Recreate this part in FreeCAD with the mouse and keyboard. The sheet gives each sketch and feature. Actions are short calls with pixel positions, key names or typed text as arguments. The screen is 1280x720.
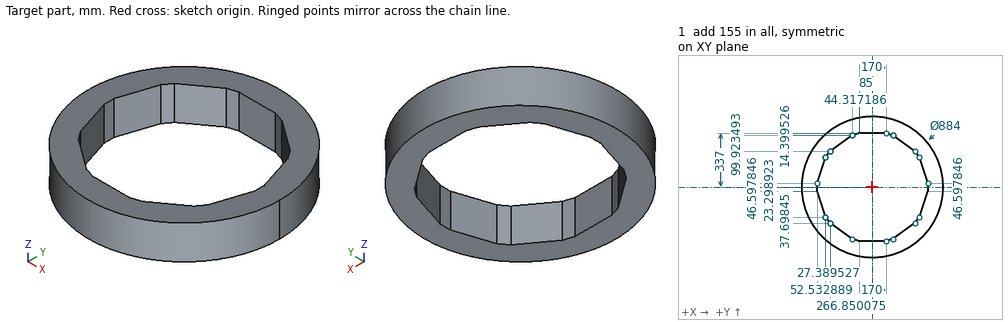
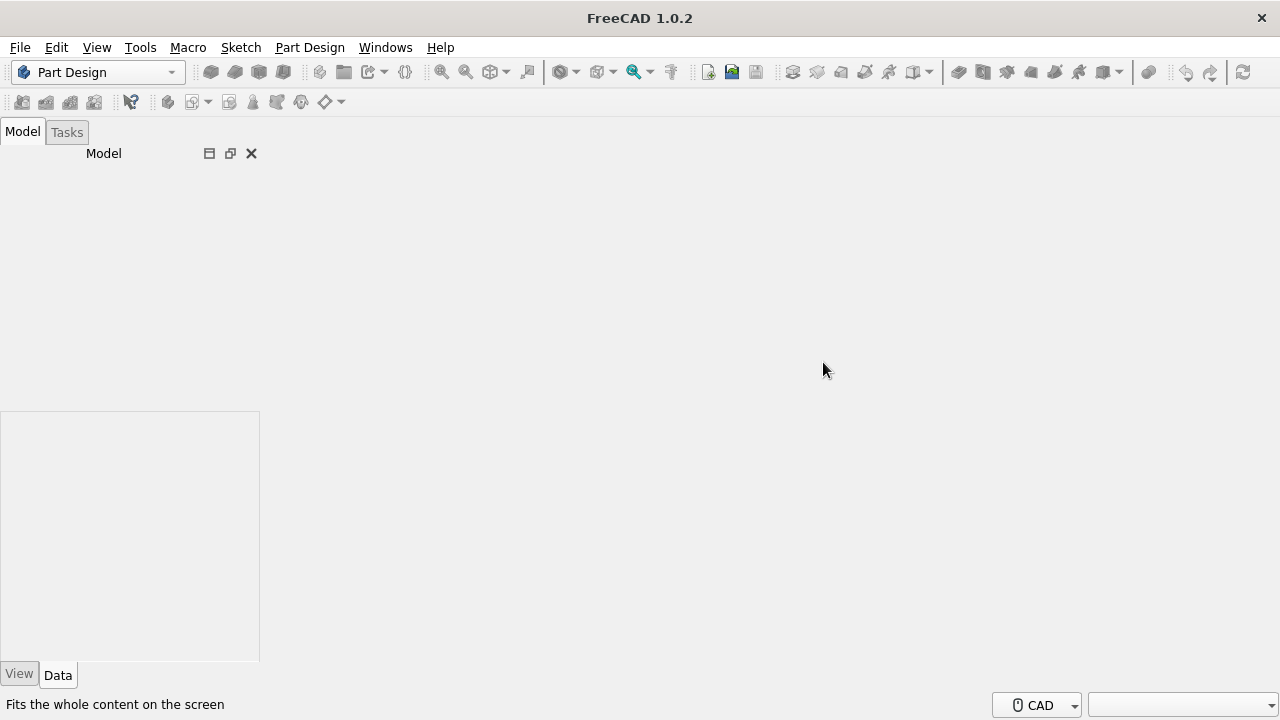
key(ctrl+n)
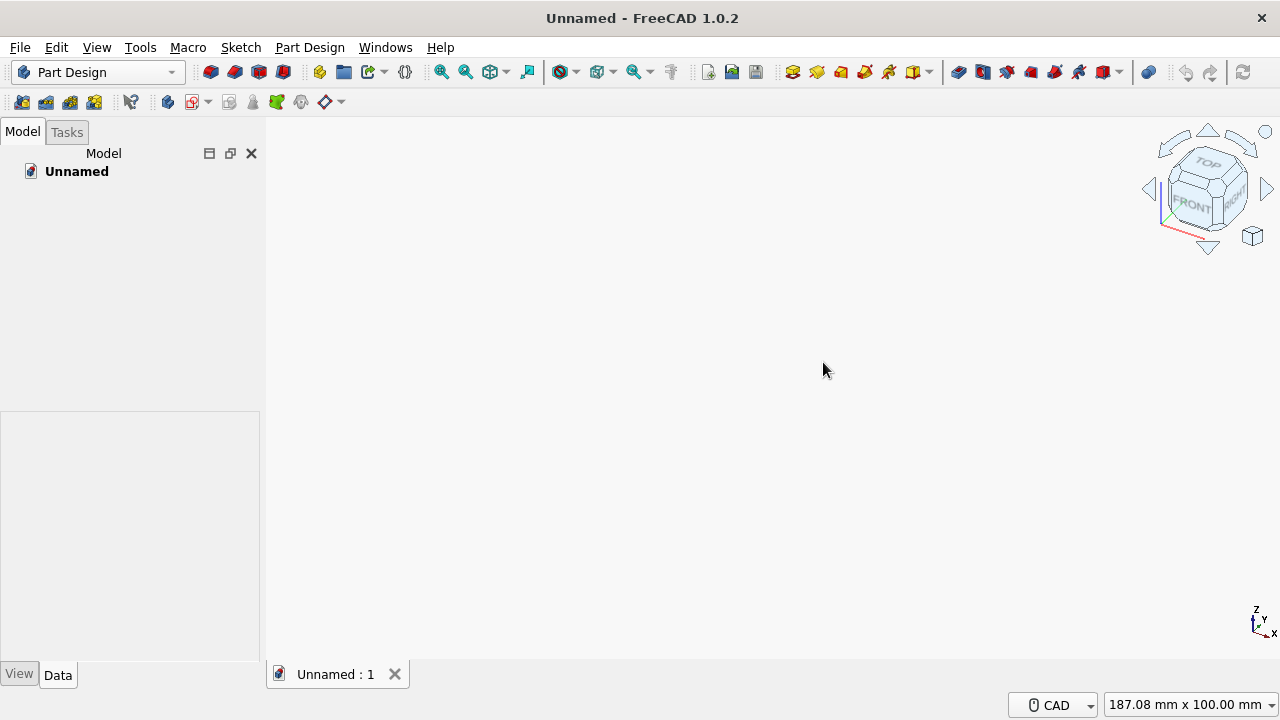
click(192, 102)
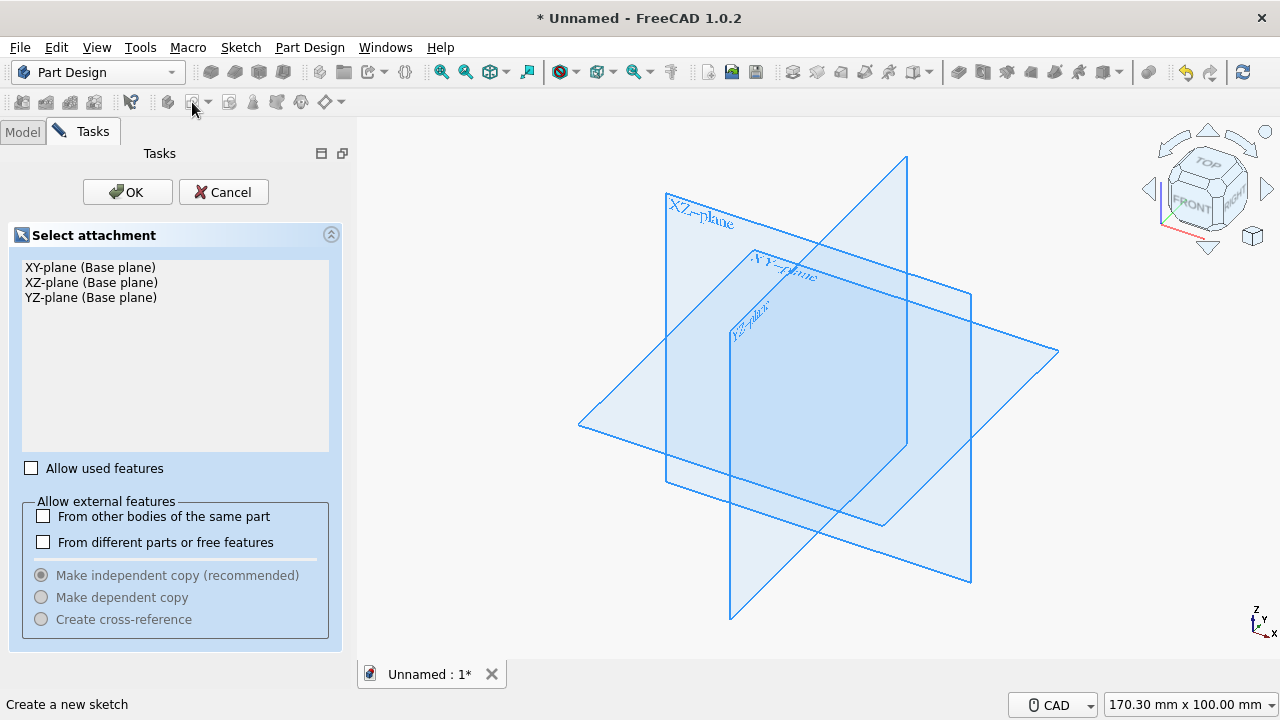
click(82, 268)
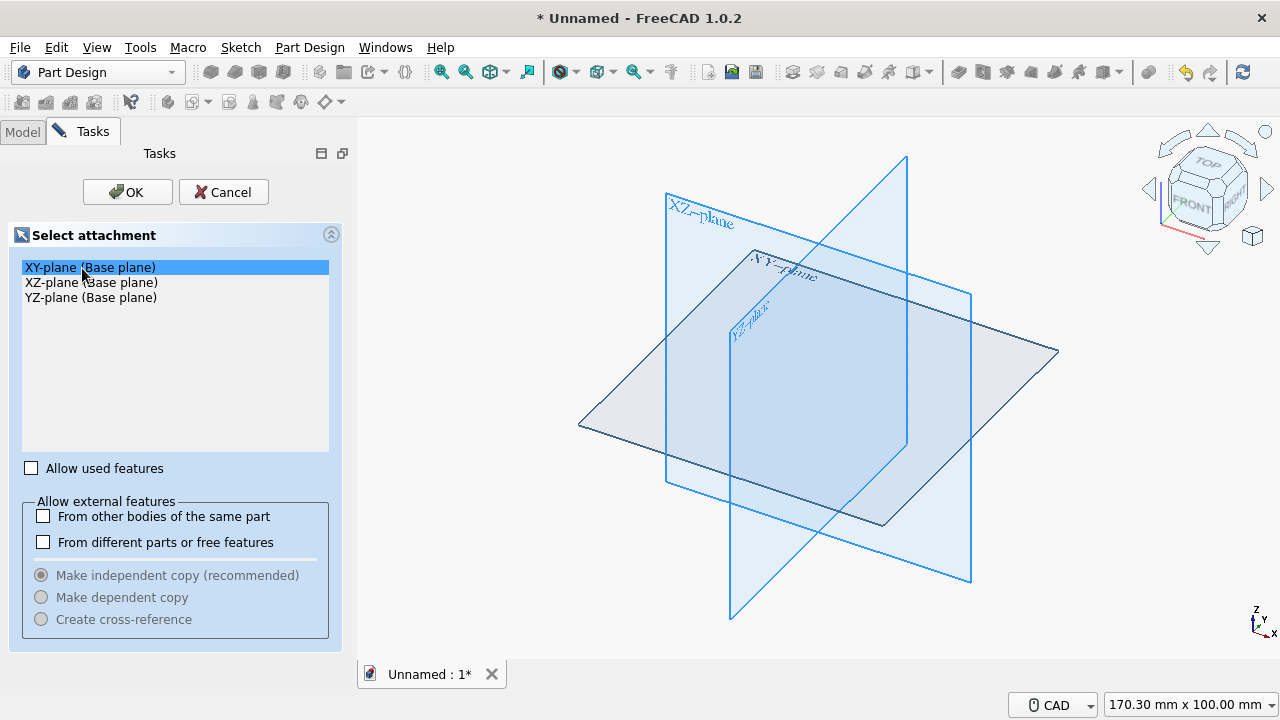
click(128, 192)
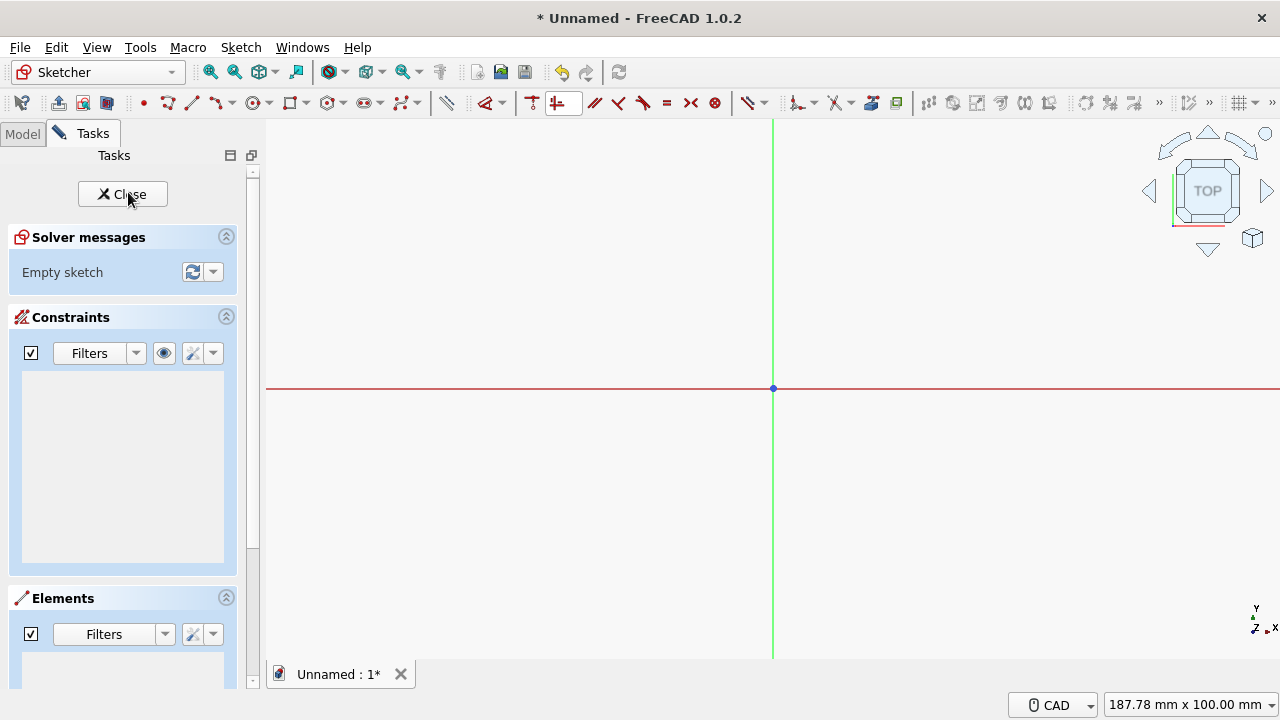
scroll(699, 389, down, 13)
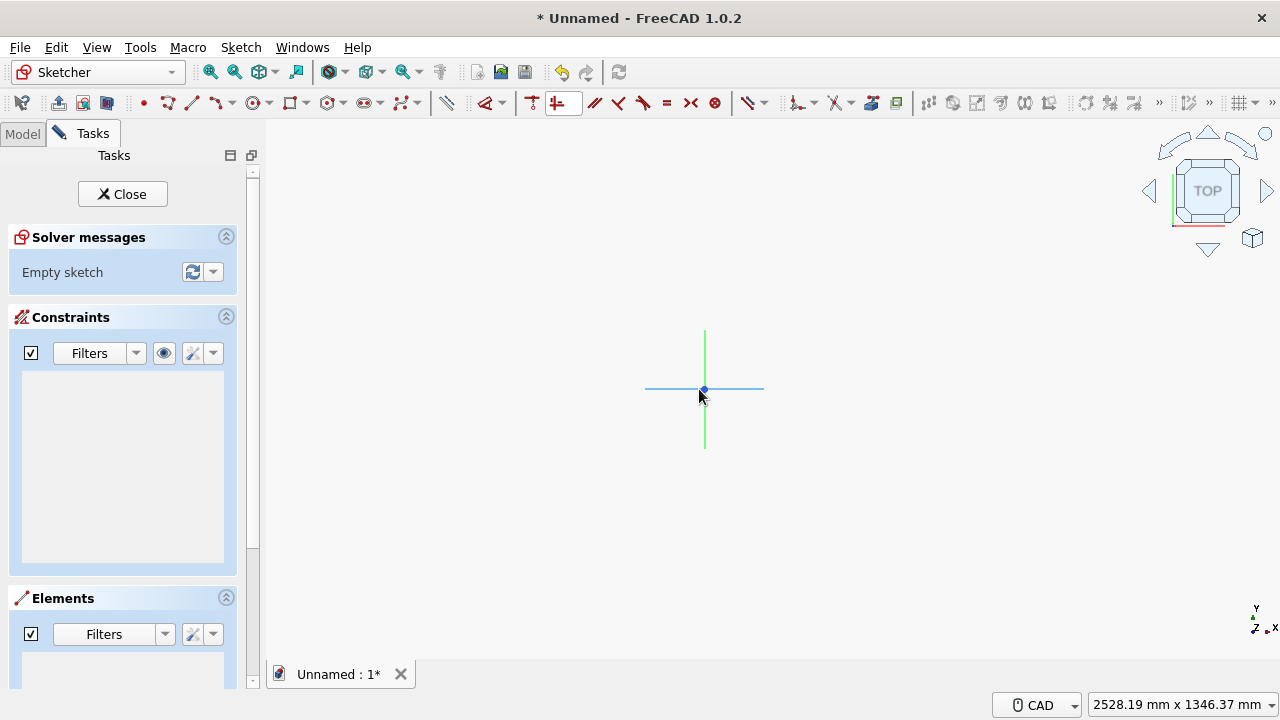
key(g)
key(m)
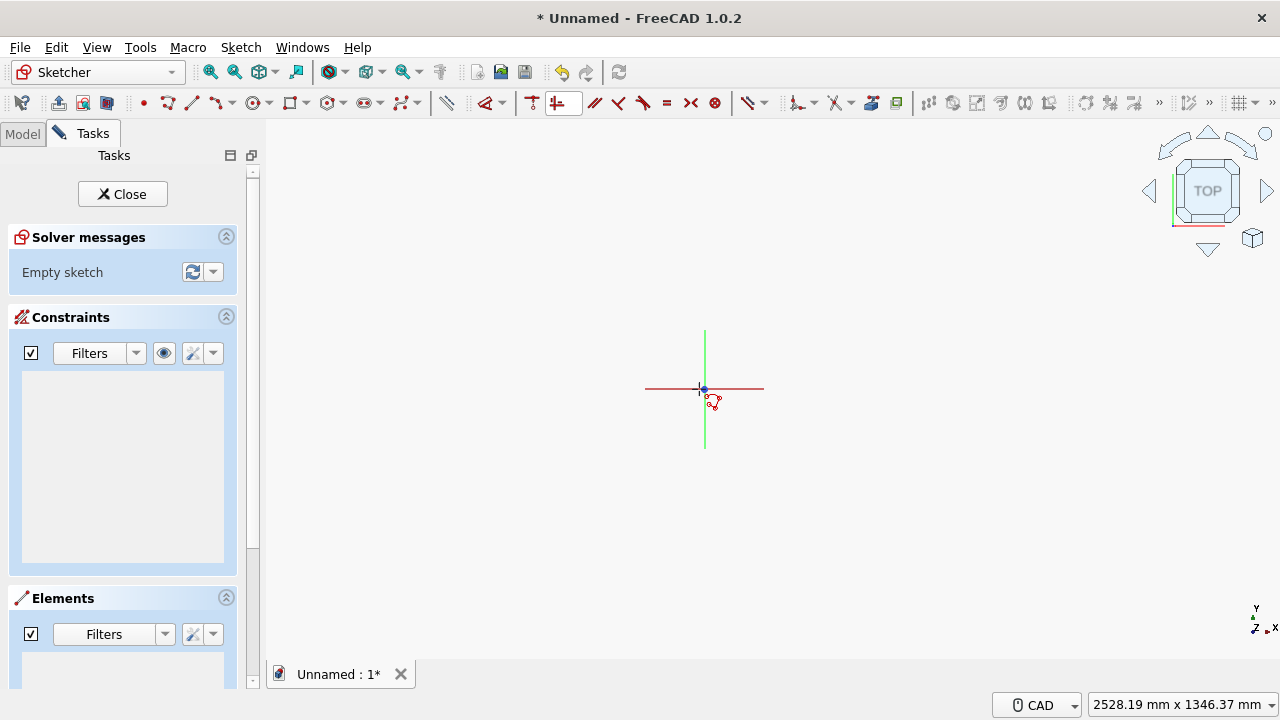
click(598, 479)
click(587, 464)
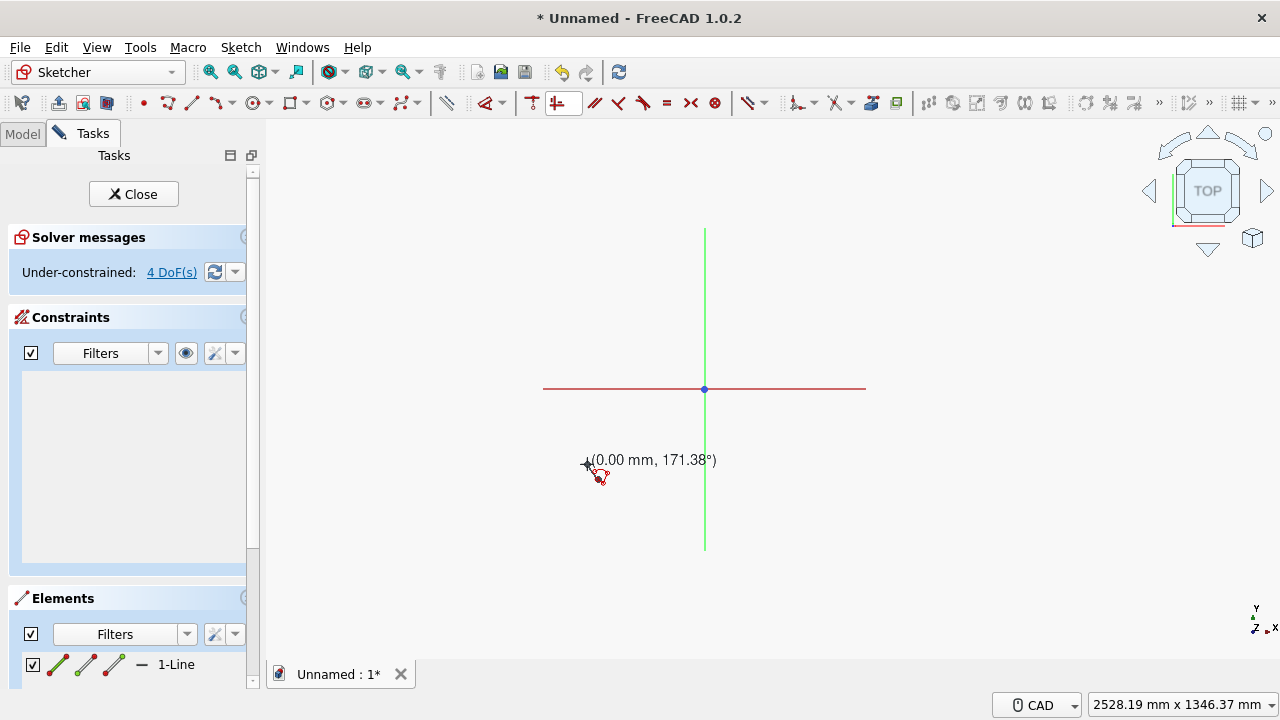
scroll(566, 399, up, 3)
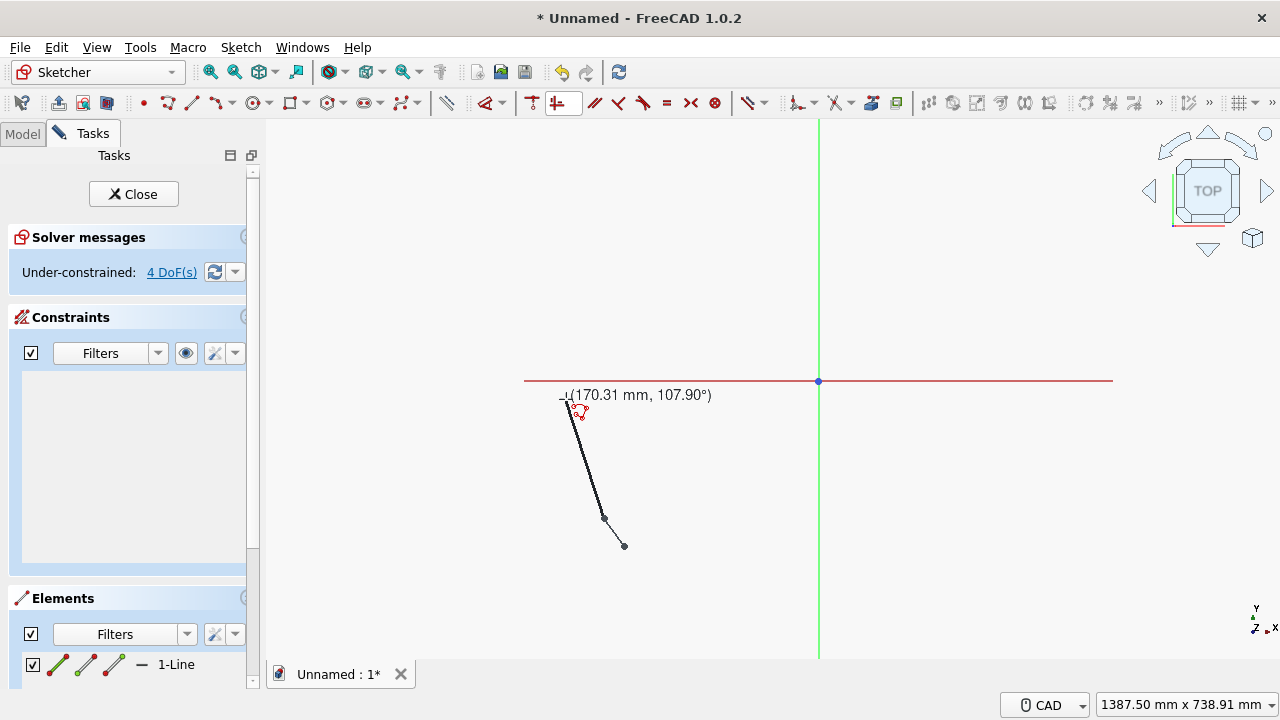
click(565, 398)
click(565, 364)
click(604, 246)
click(624, 218)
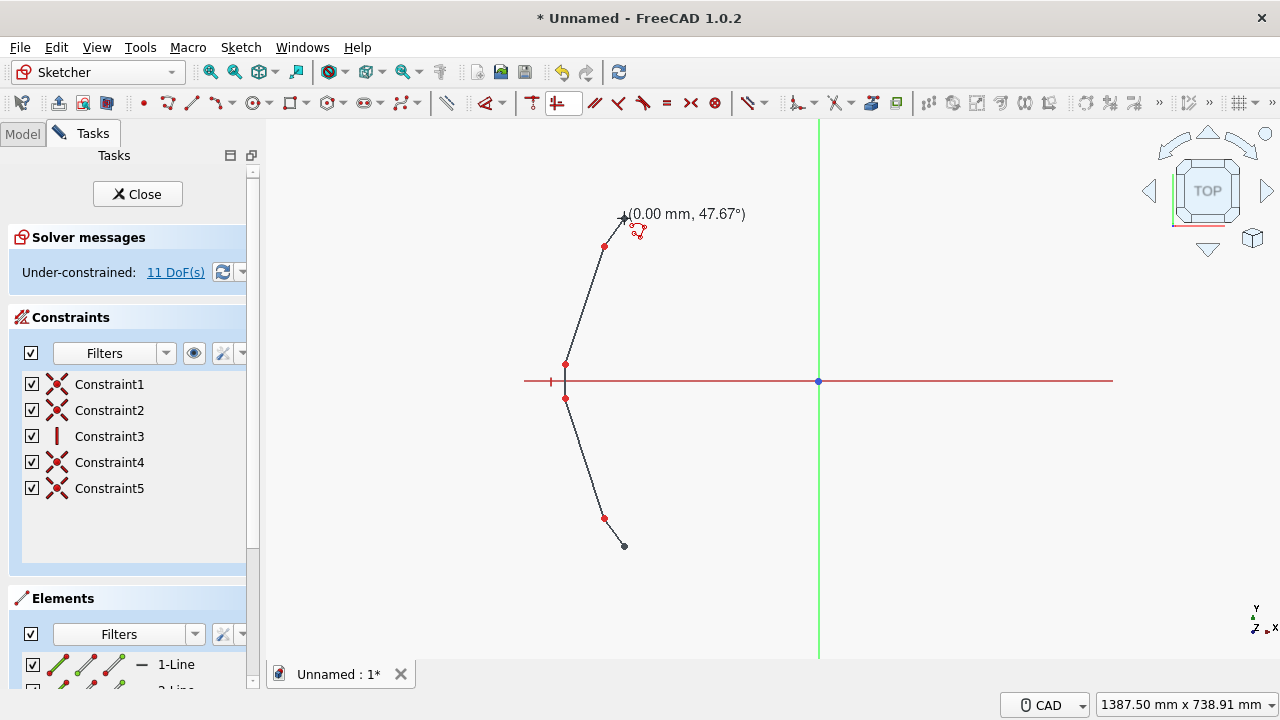
scroll(565, 398, down, 3)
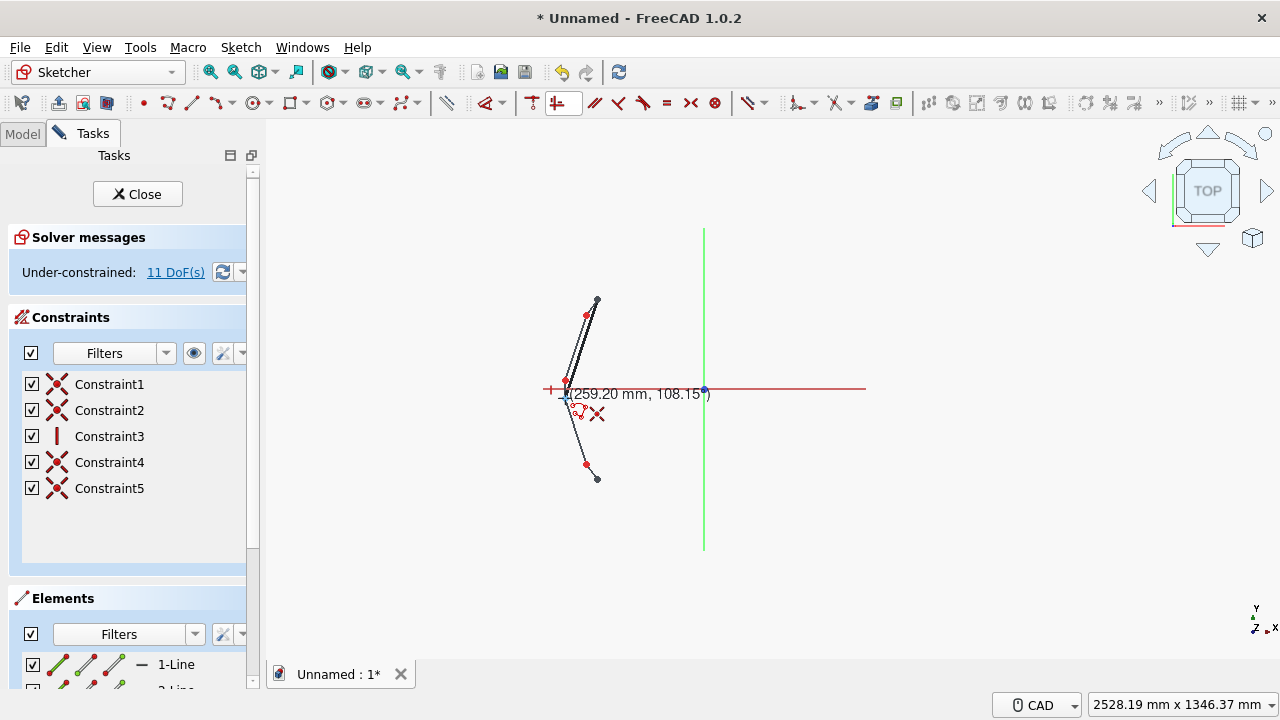
click(653, 260)
click(670, 254)
click(739, 254)
click(756, 260)
click(811, 300)
click(822, 315)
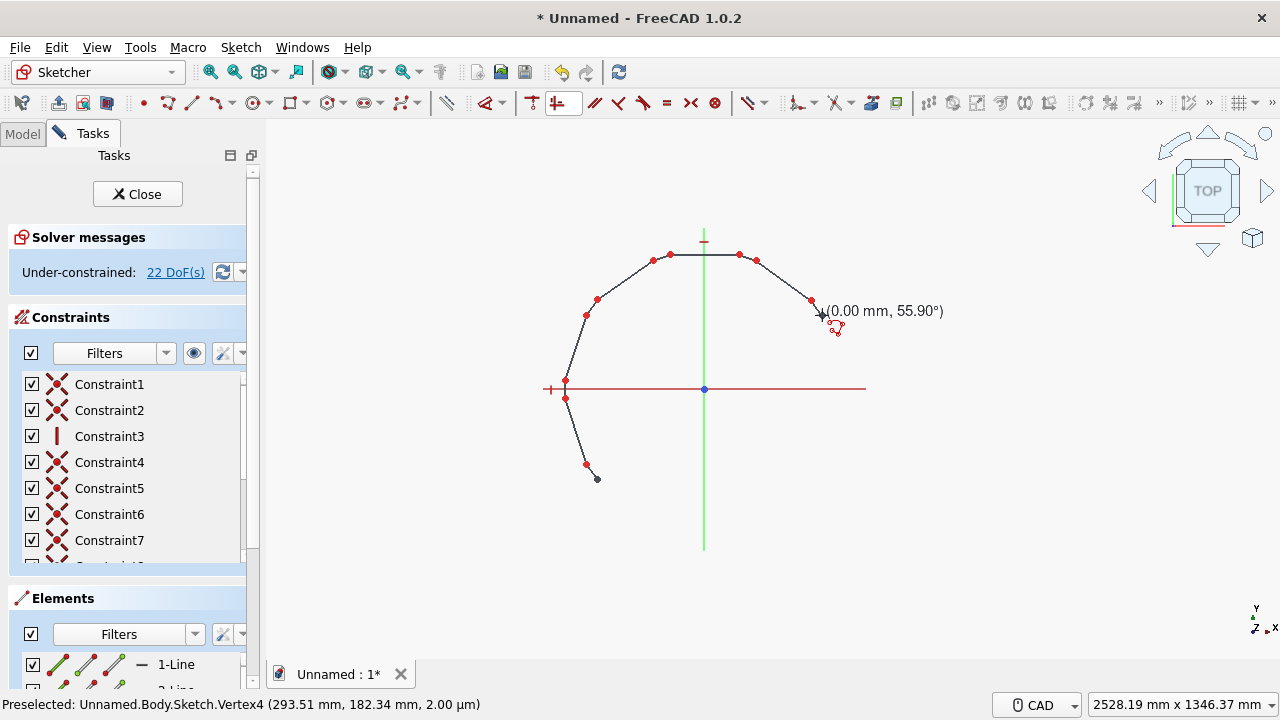
scroll(844, 380, up, 3)